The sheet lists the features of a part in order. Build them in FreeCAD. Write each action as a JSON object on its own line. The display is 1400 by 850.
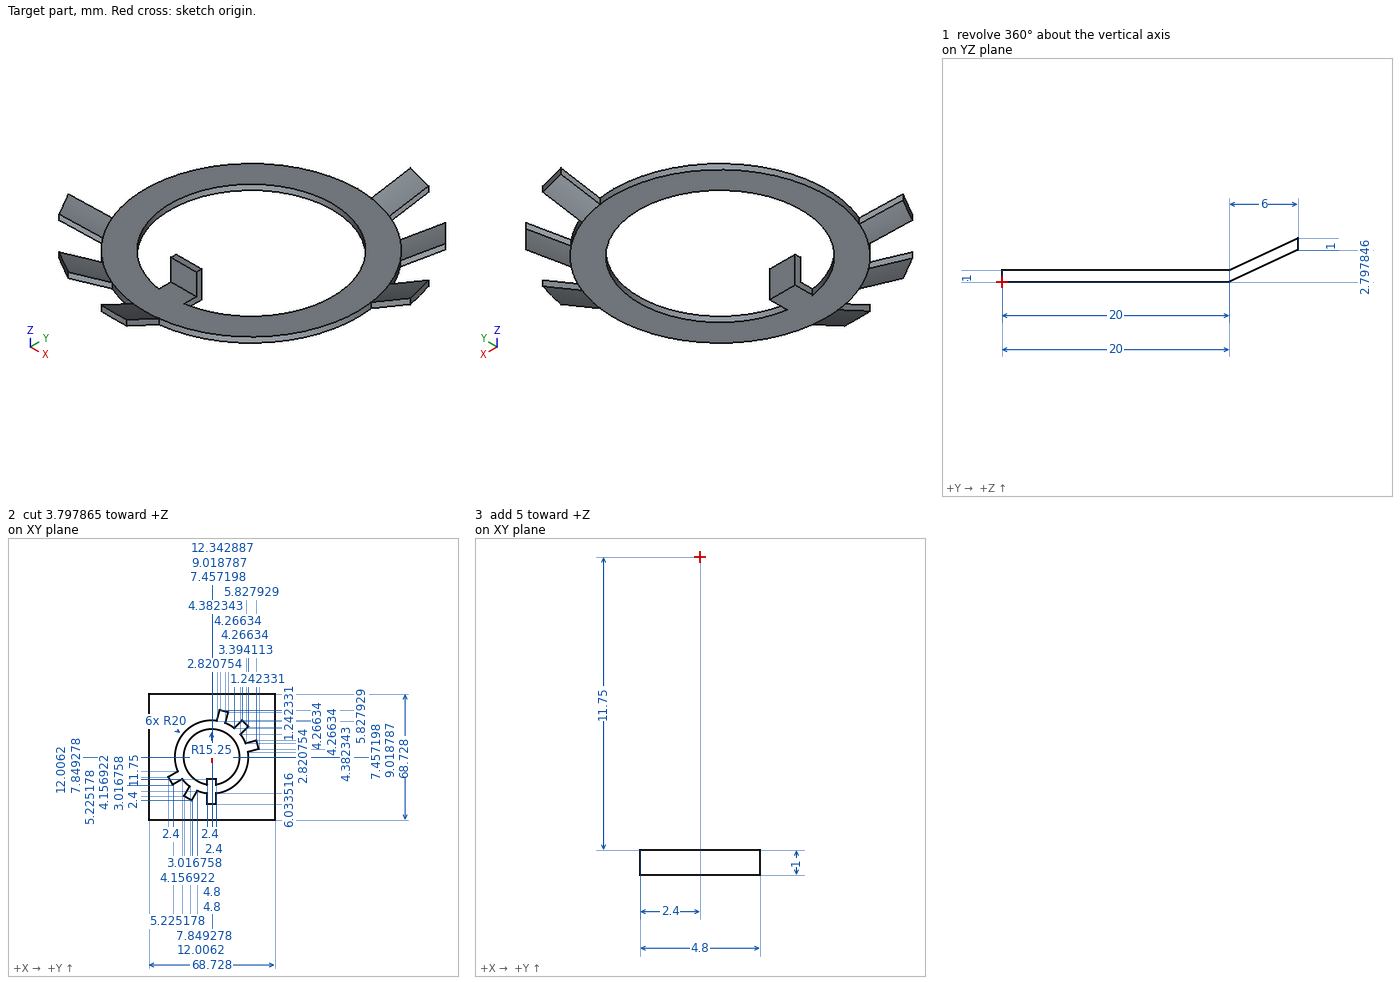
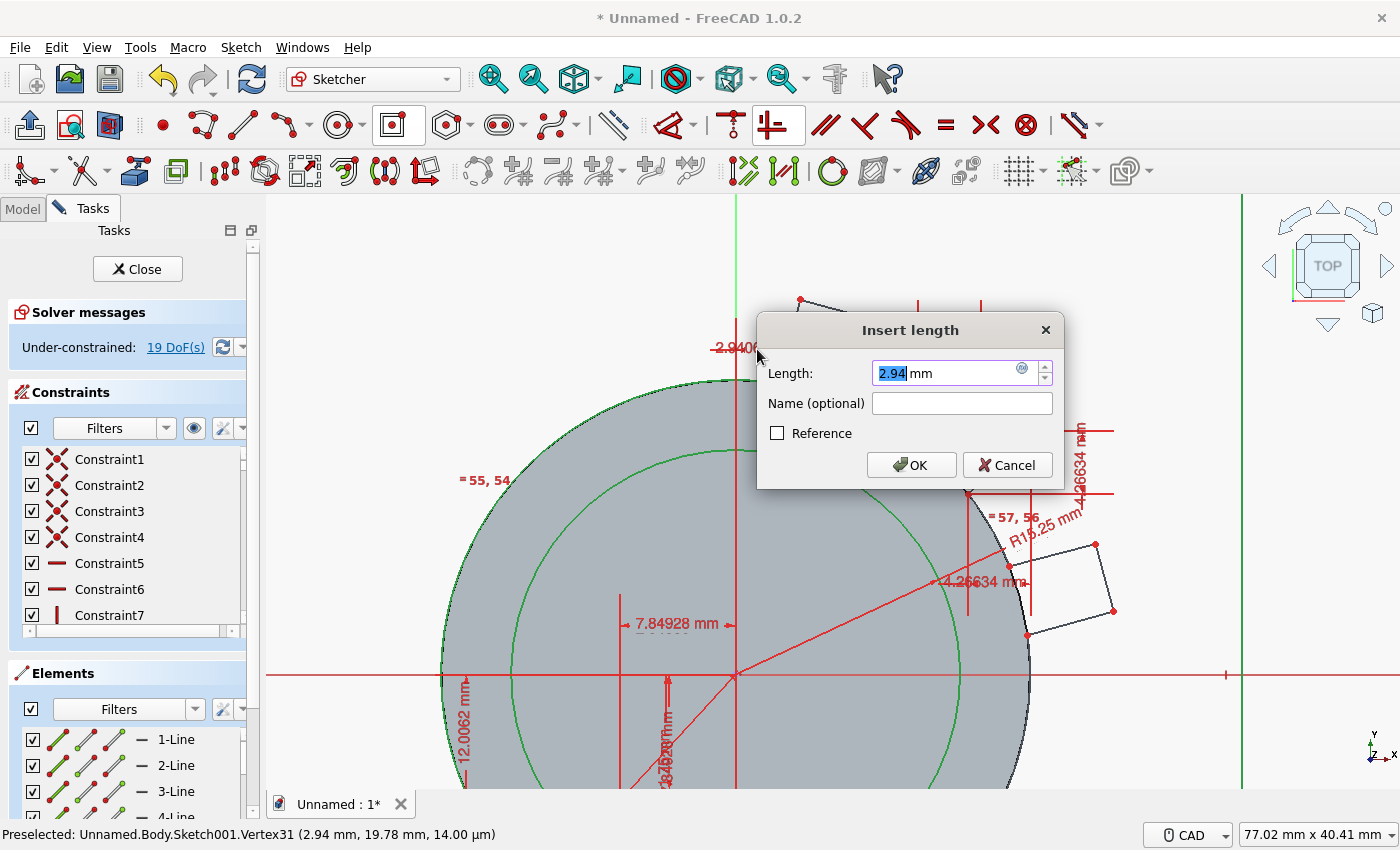
{"action": "type", "text": "2.820754"}
{"action": "key", "text": "Return"}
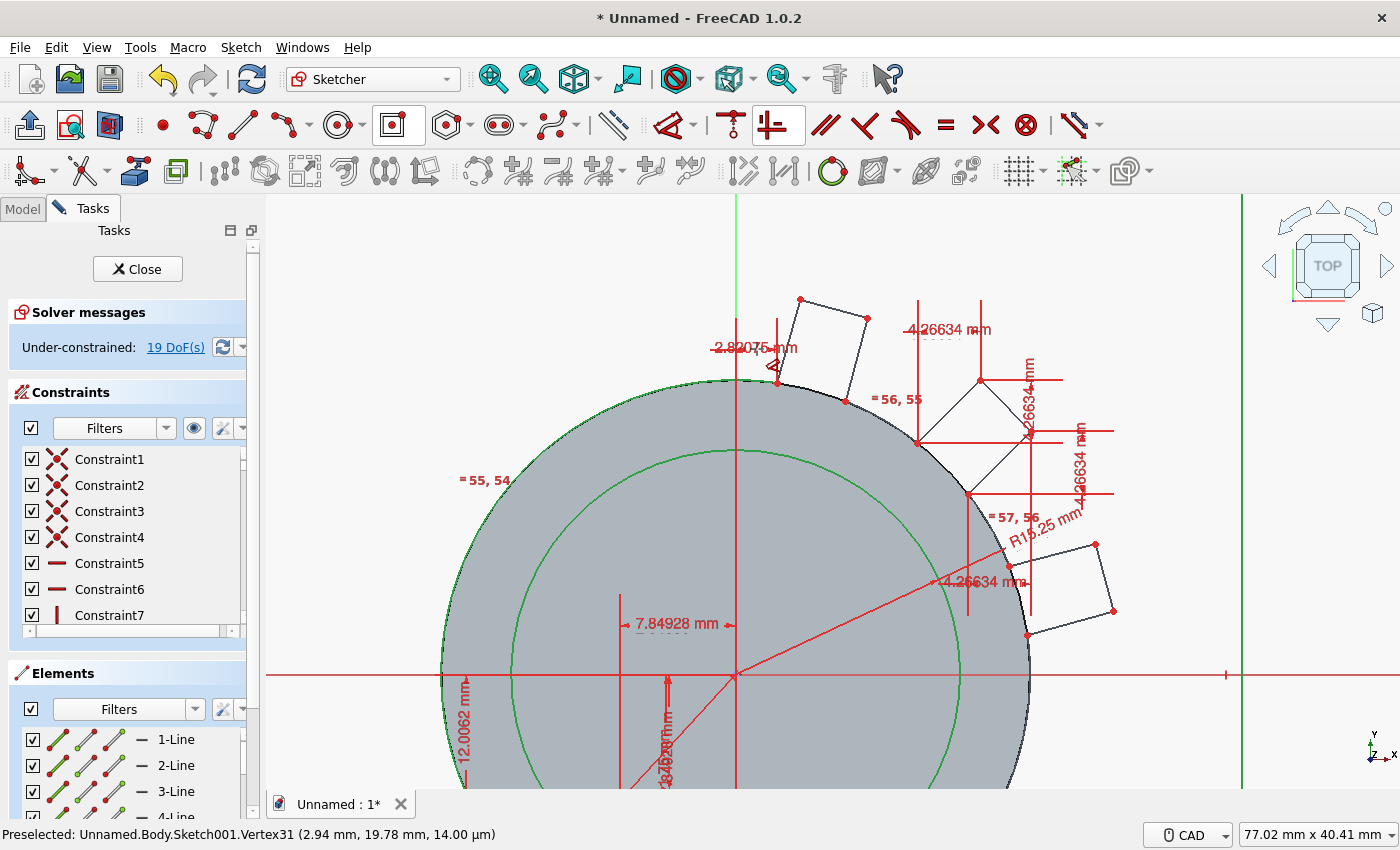
{"action": "left_click", "coordinate": [800, 300]}
{"action": "left_click", "coordinate": [768, 266]}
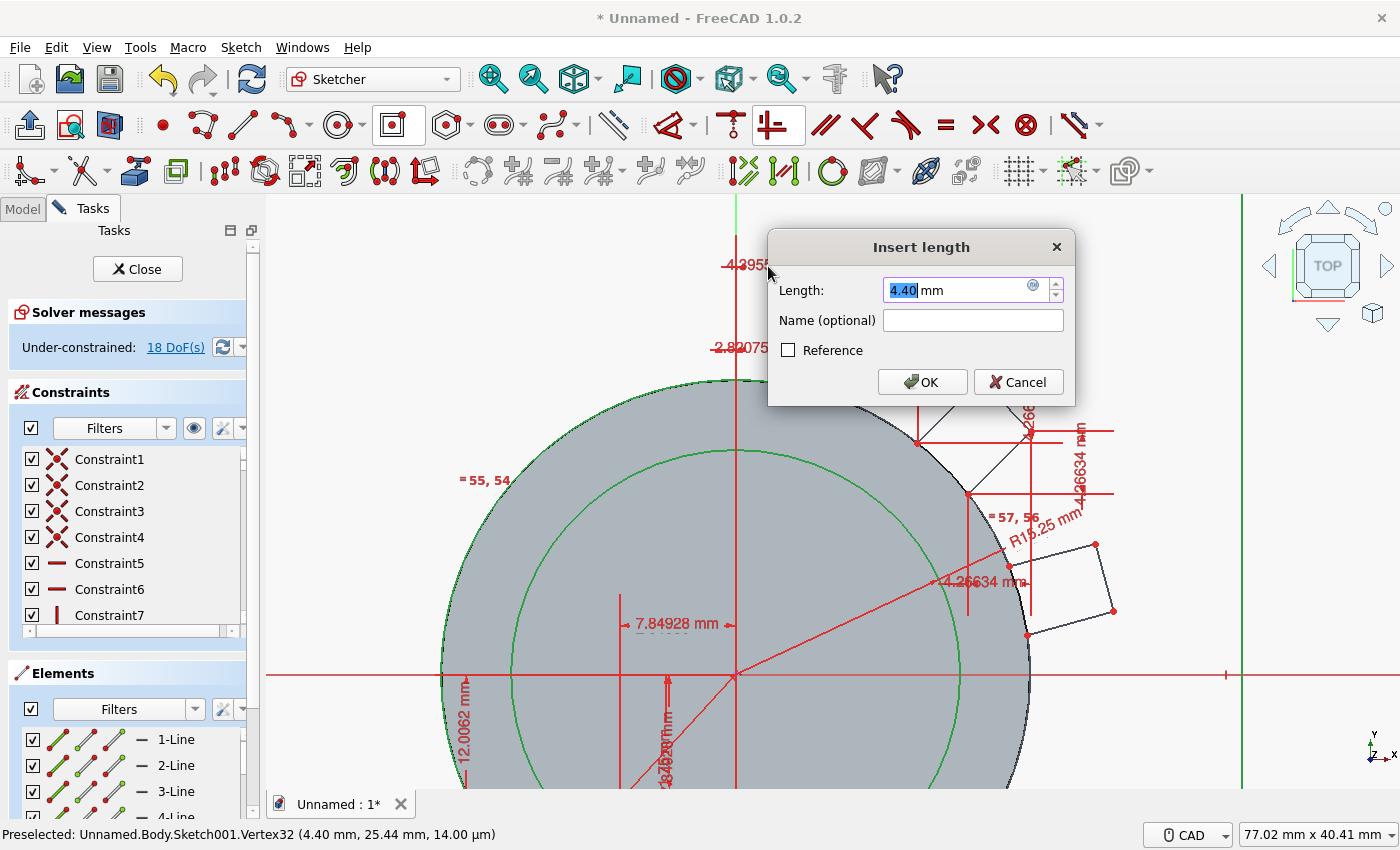
{"action": "type", "text": "4.382343"}
{"action": "key", "text": "Return"}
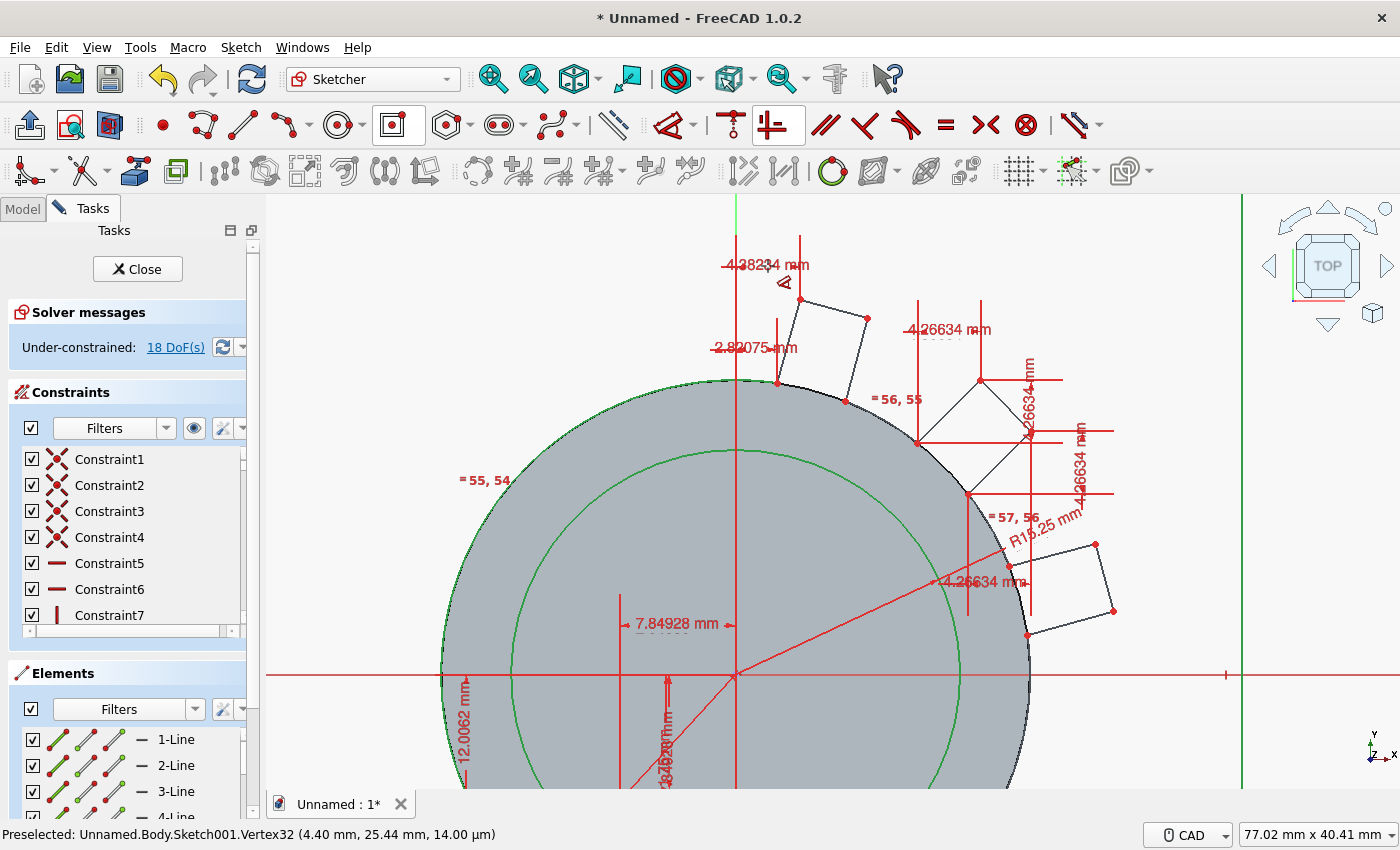
{"action": "left_click", "coordinate": [868, 318]}
{"action": "left_click", "coordinate": [848, 284]}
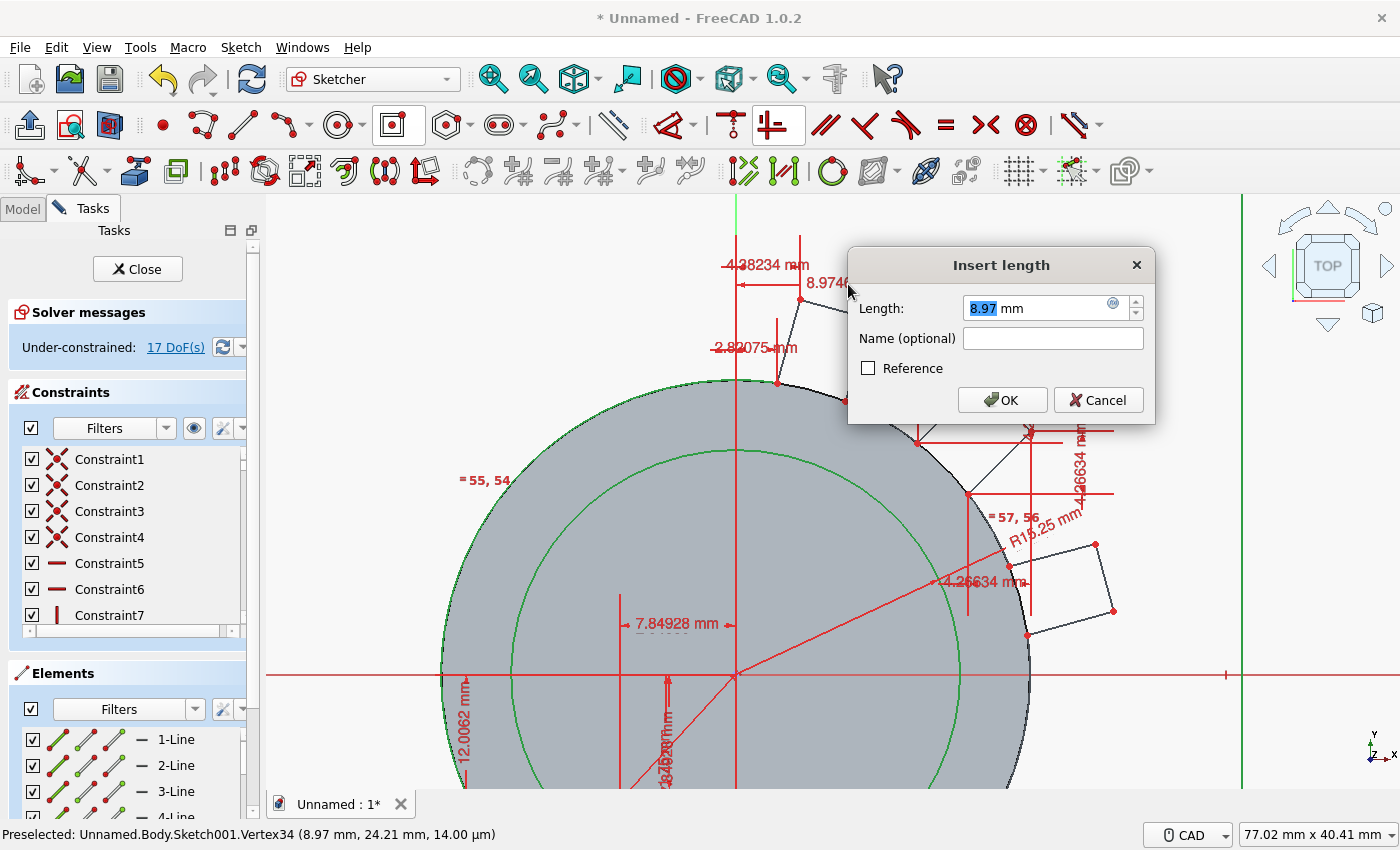
{"action": "type", "text": "9.018787"}
{"action": "key", "text": "Return"}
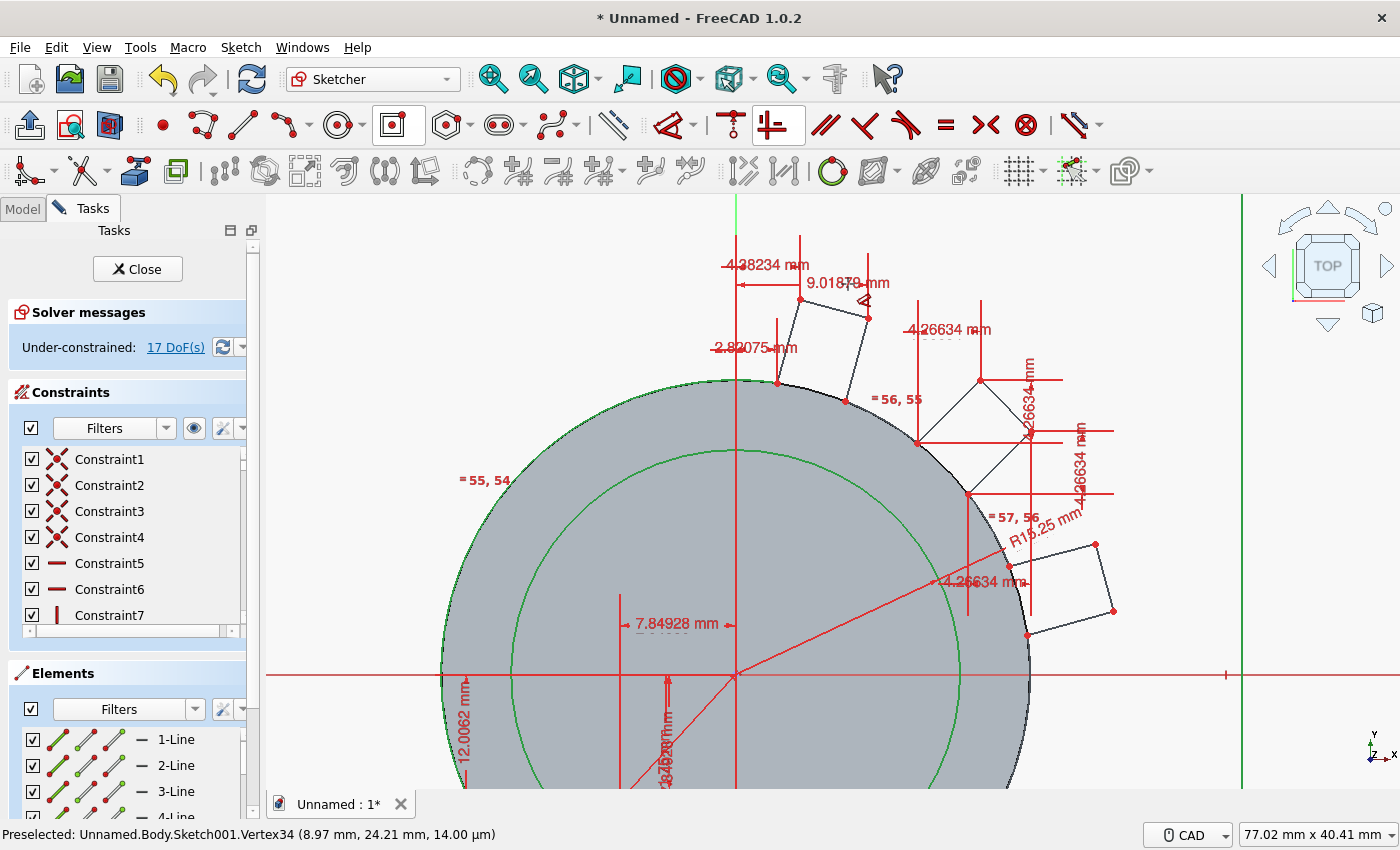
{"action": "left_click", "coordinate": [846, 401]}
{"action": "left_click", "coordinate": [829, 367]}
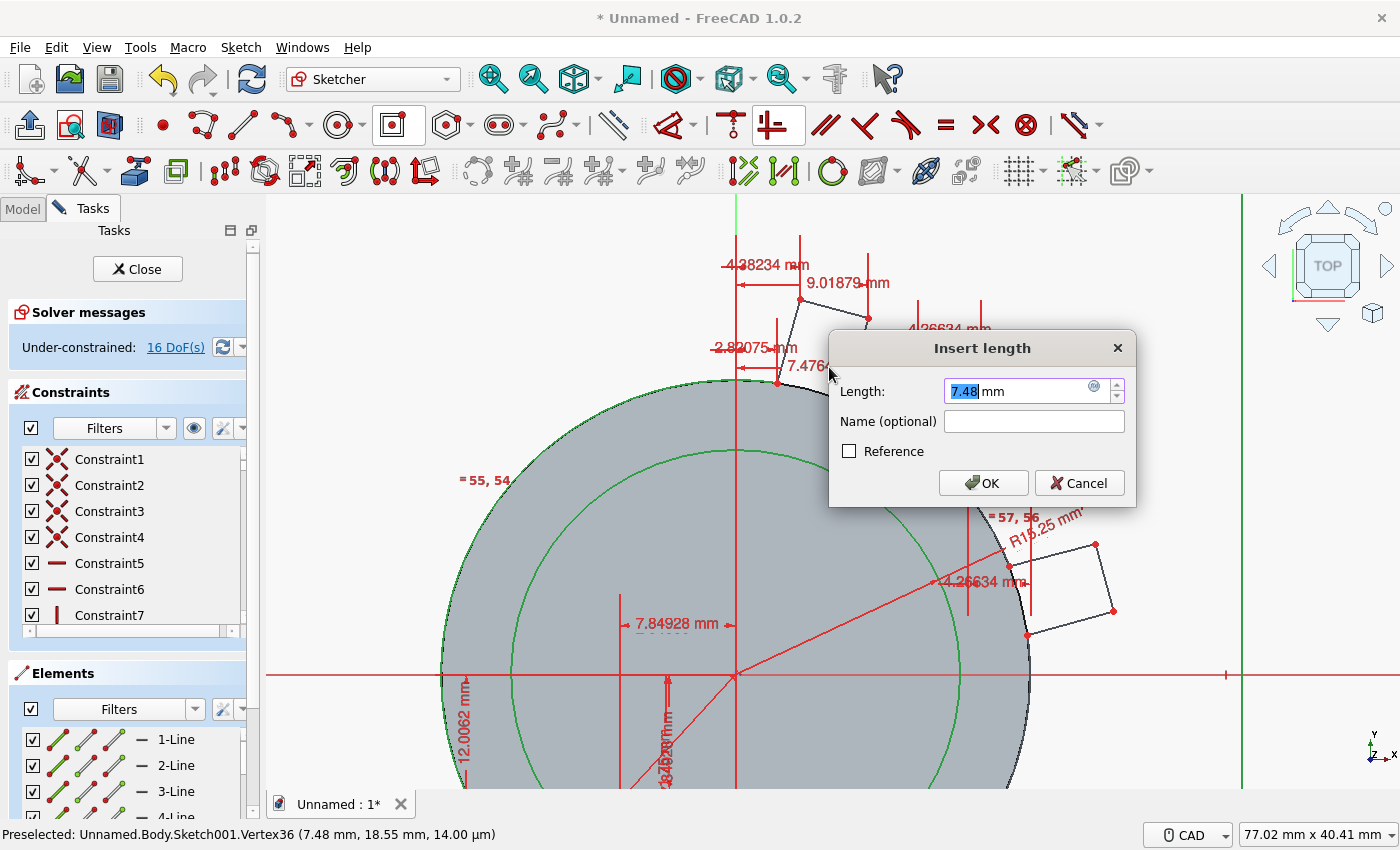
{"action": "type", "text": "7.457198"}
{"action": "key", "text": "Return"}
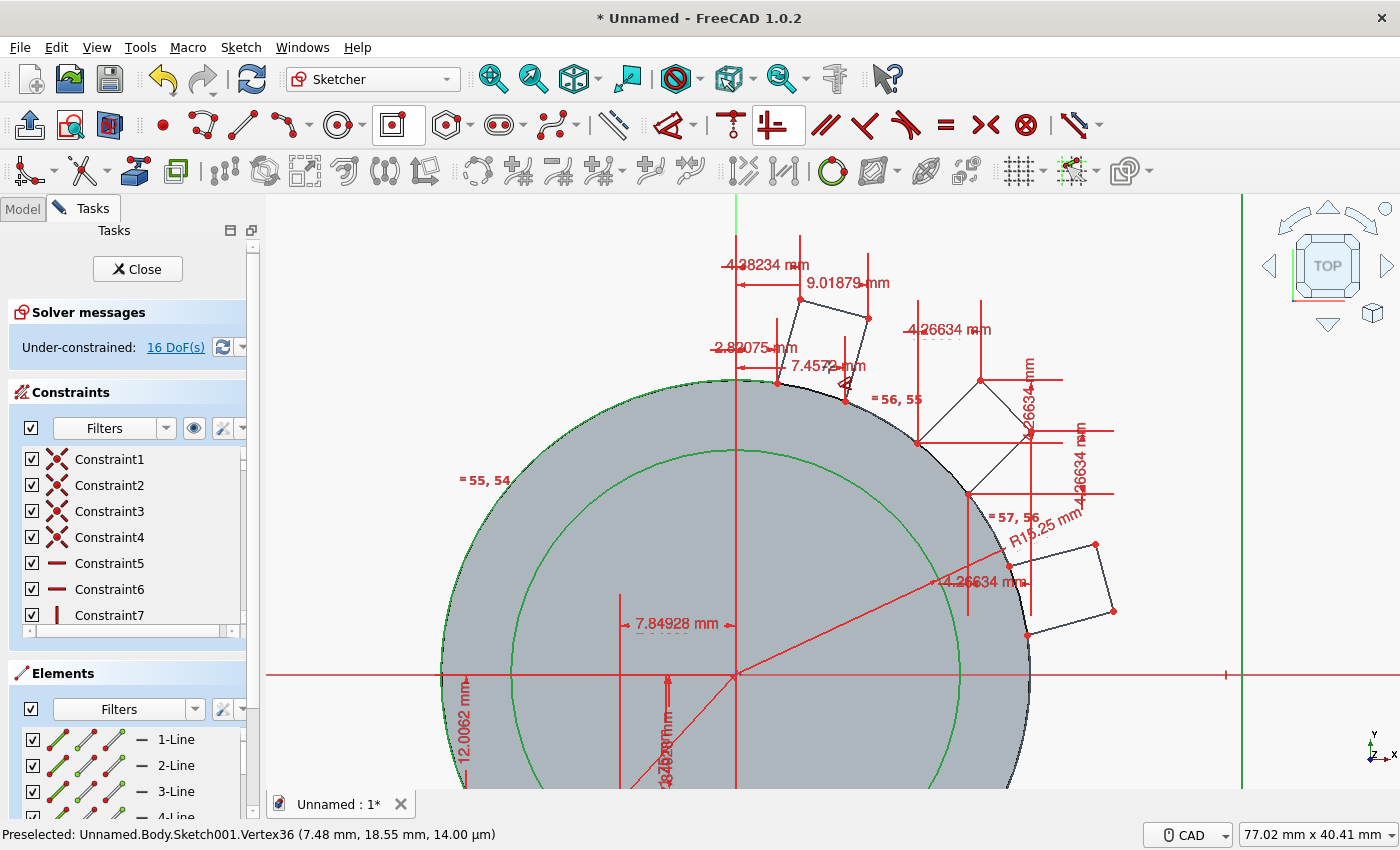
{"action": "left_click", "coordinate": [1010, 566]}
{"action": "left_click", "coordinate": [1044, 645]}